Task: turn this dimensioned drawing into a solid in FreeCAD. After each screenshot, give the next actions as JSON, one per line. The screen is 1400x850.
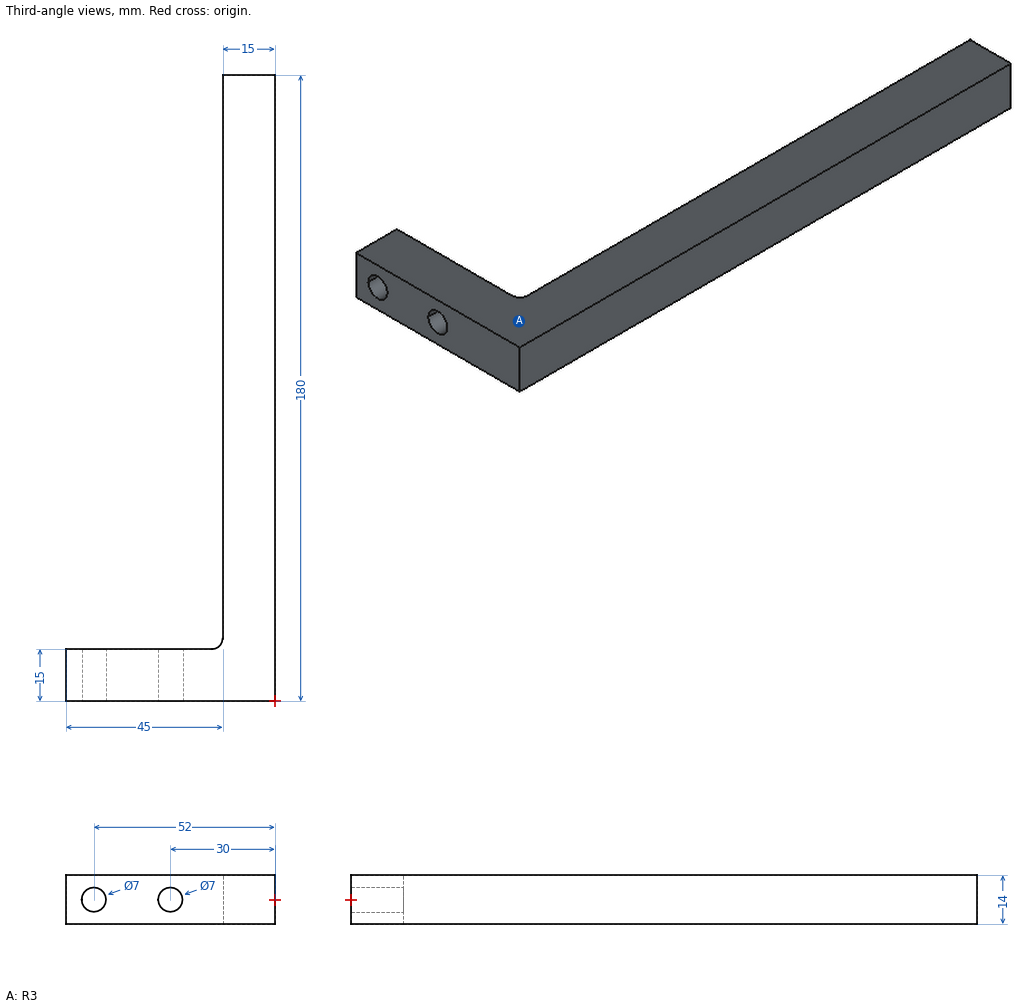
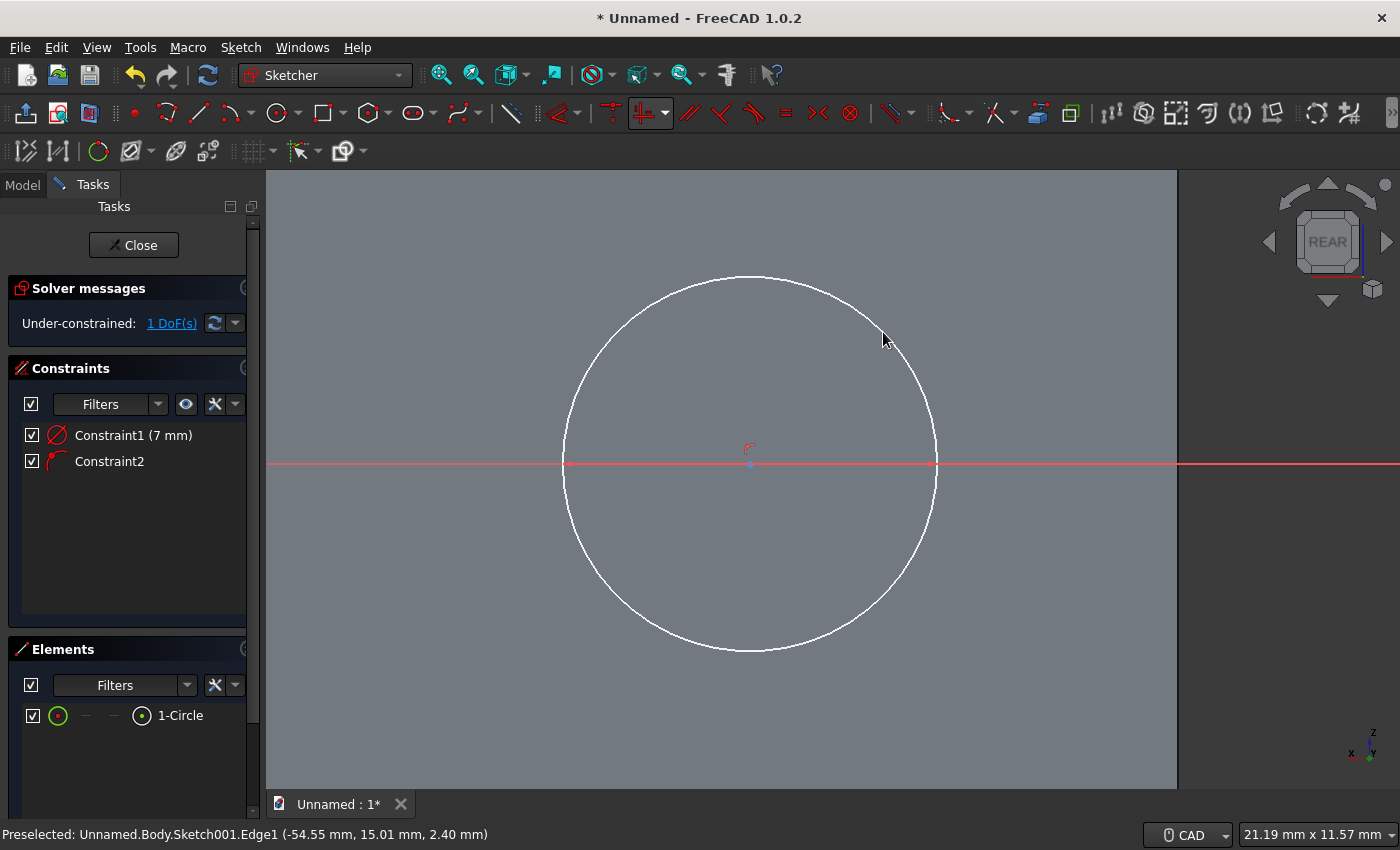
{"action": "left_click", "coordinate": [750, 464]}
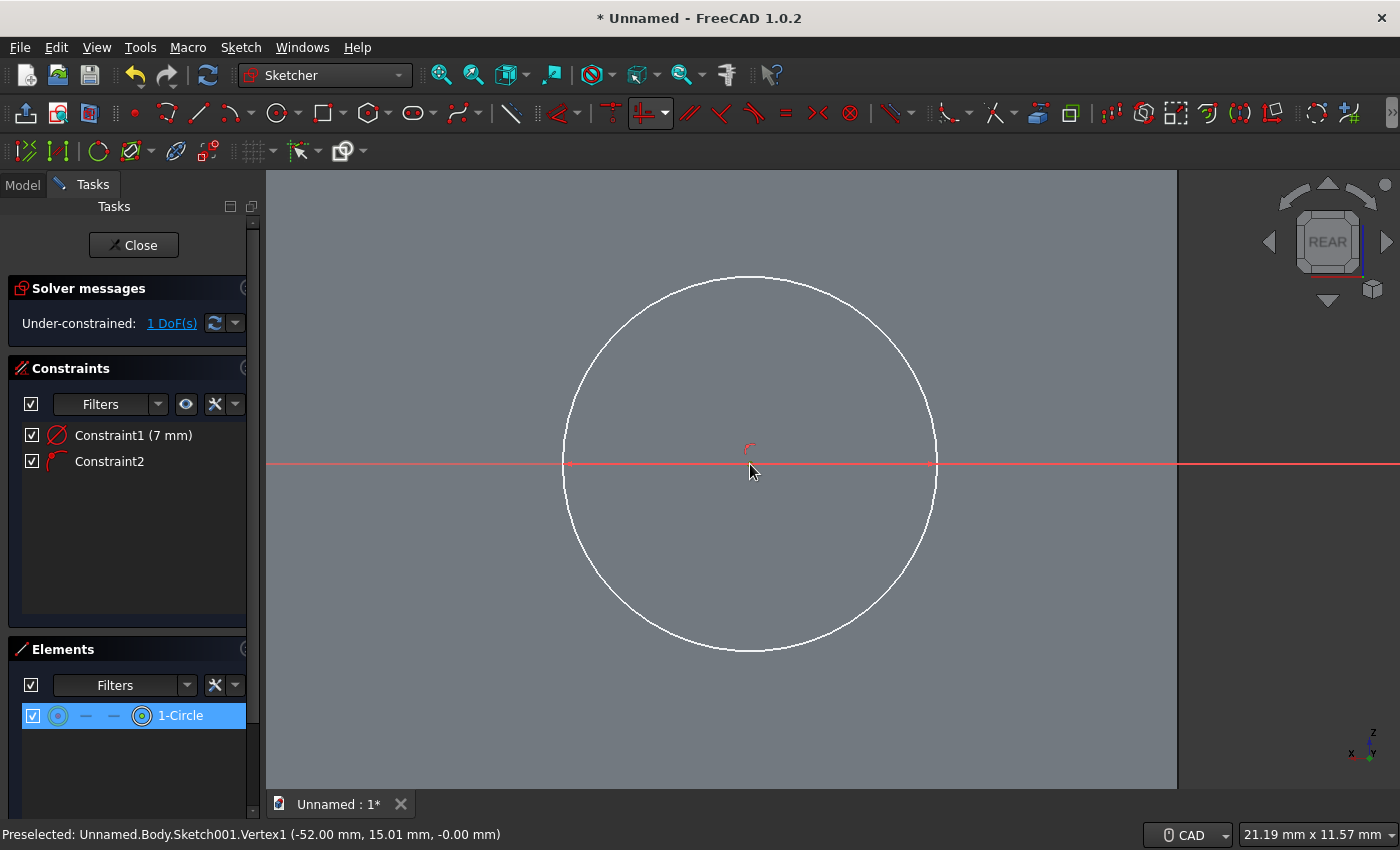
{"action": "left_click", "coordinate": [580, 114]}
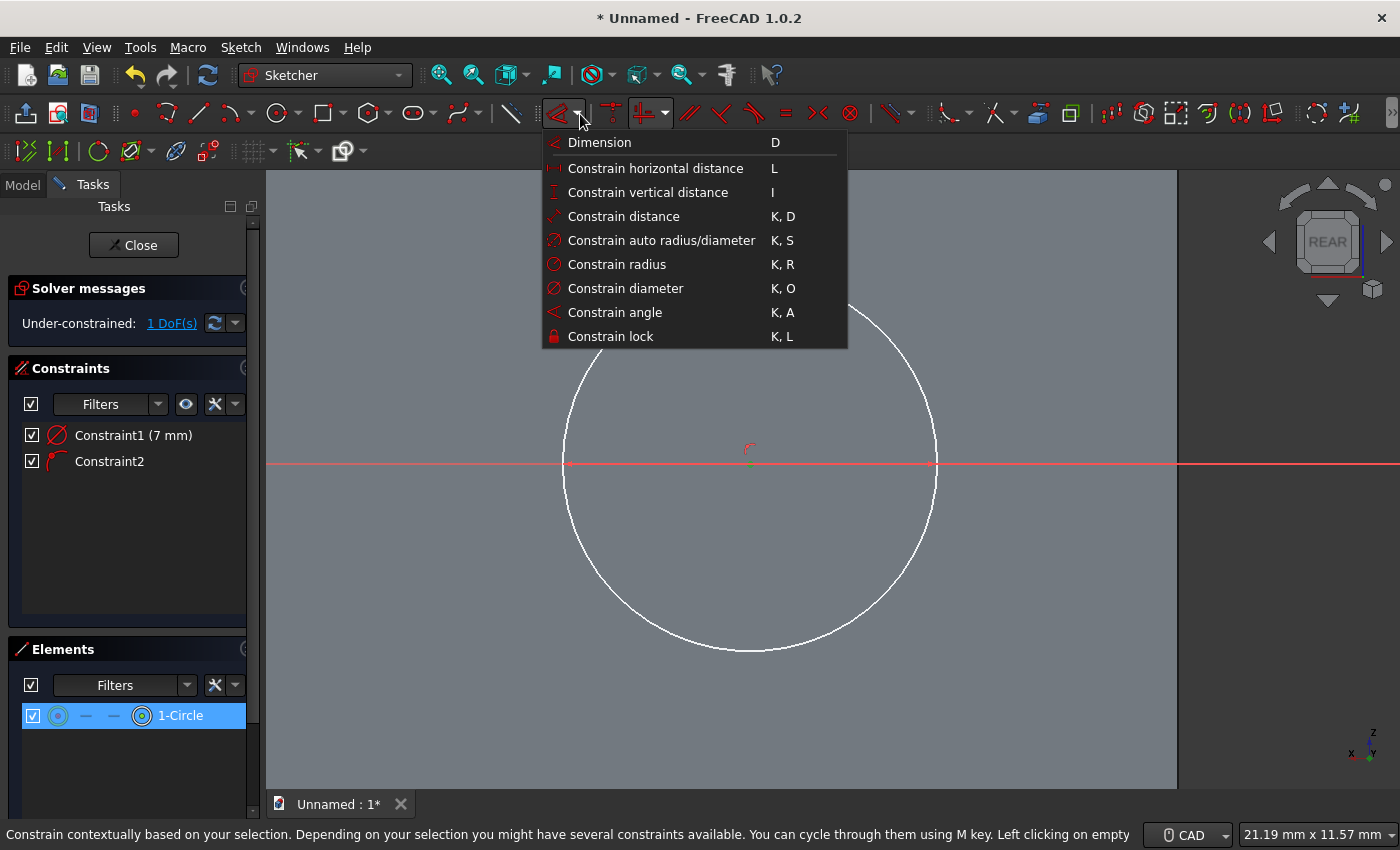
{"action": "left_click", "coordinate": [695, 168]}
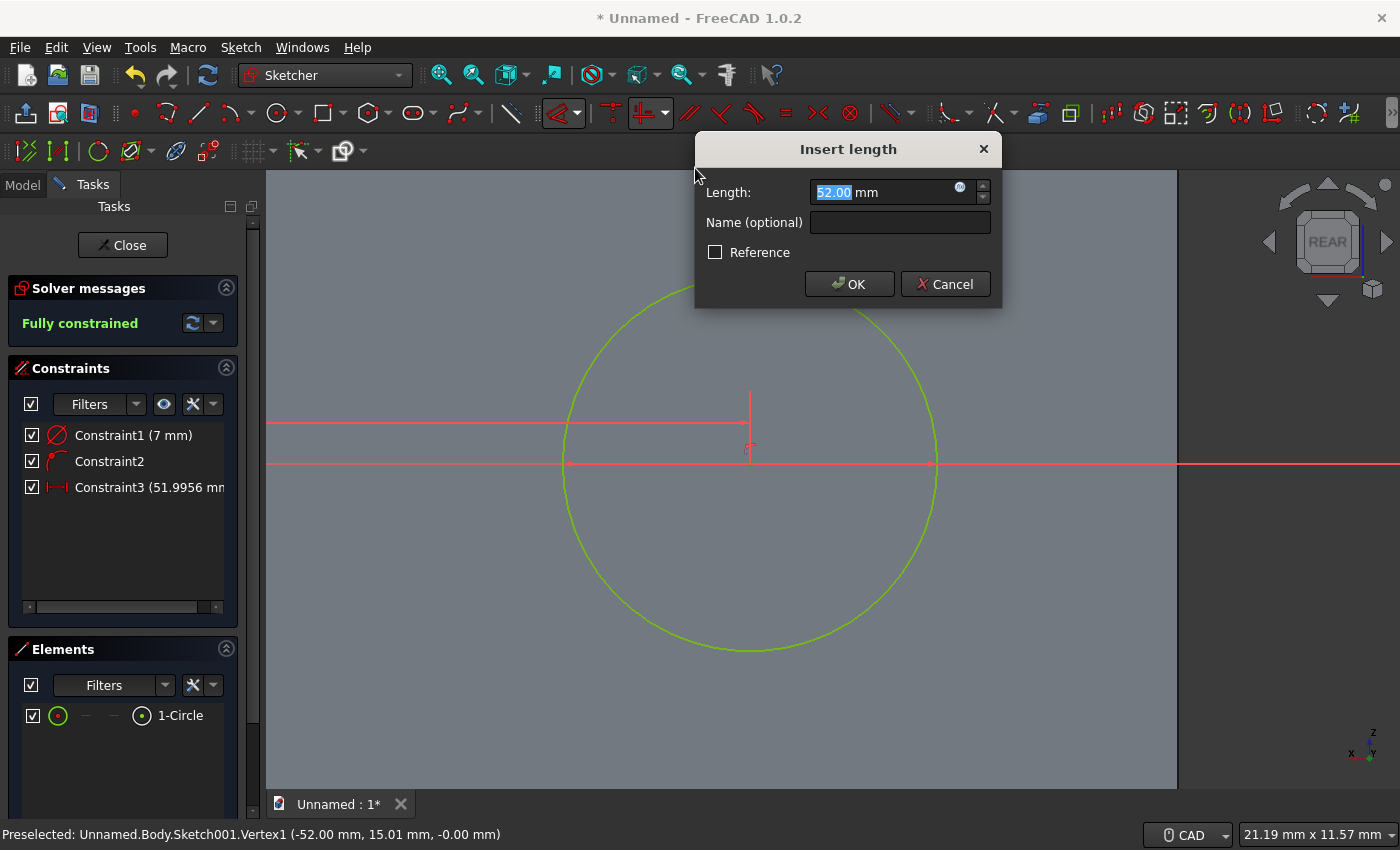
{"action": "type", "text": "52"}
{"action": "key", "text": "Return"}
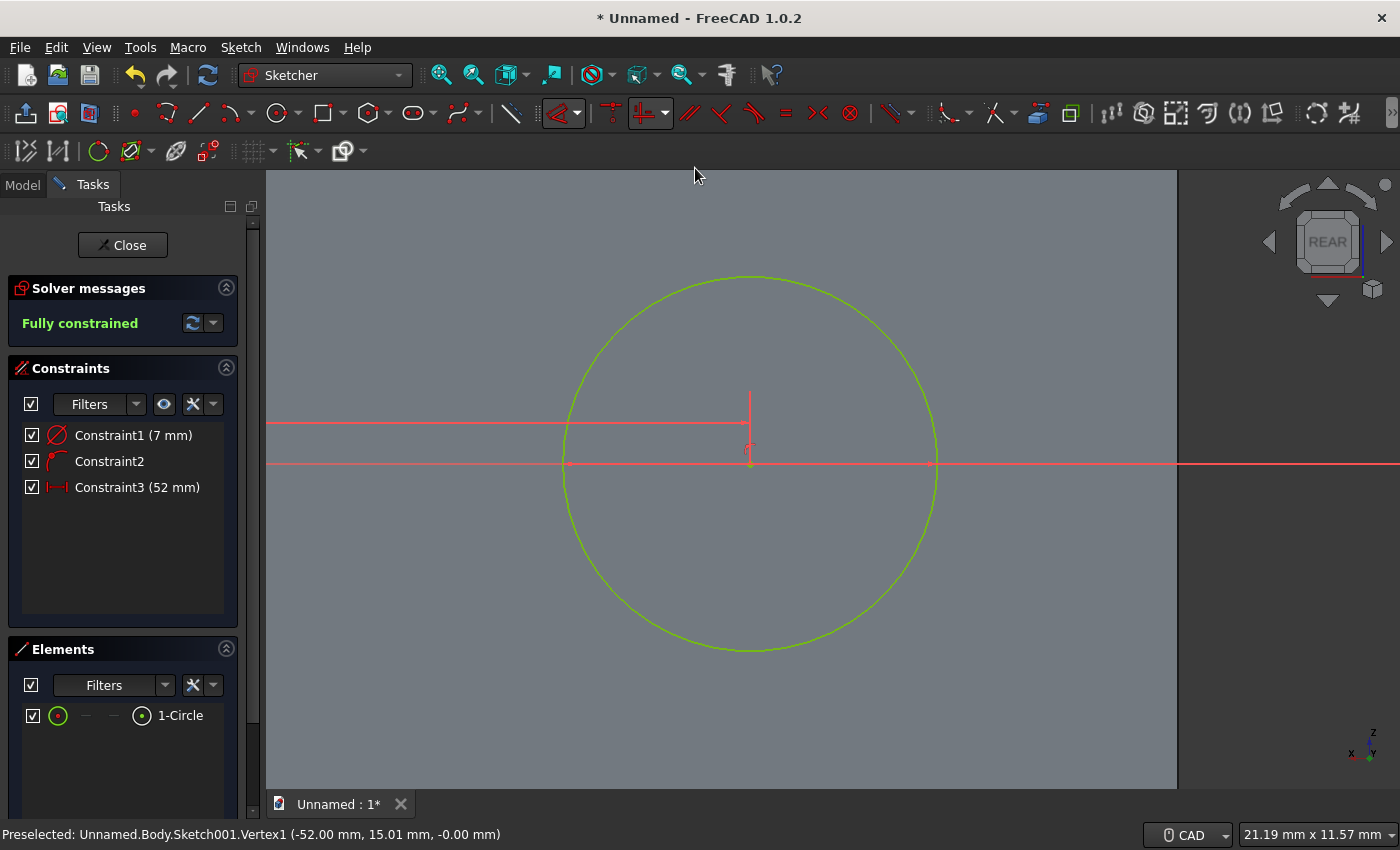
{"action": "left_click", "coordinate": [123, 245]}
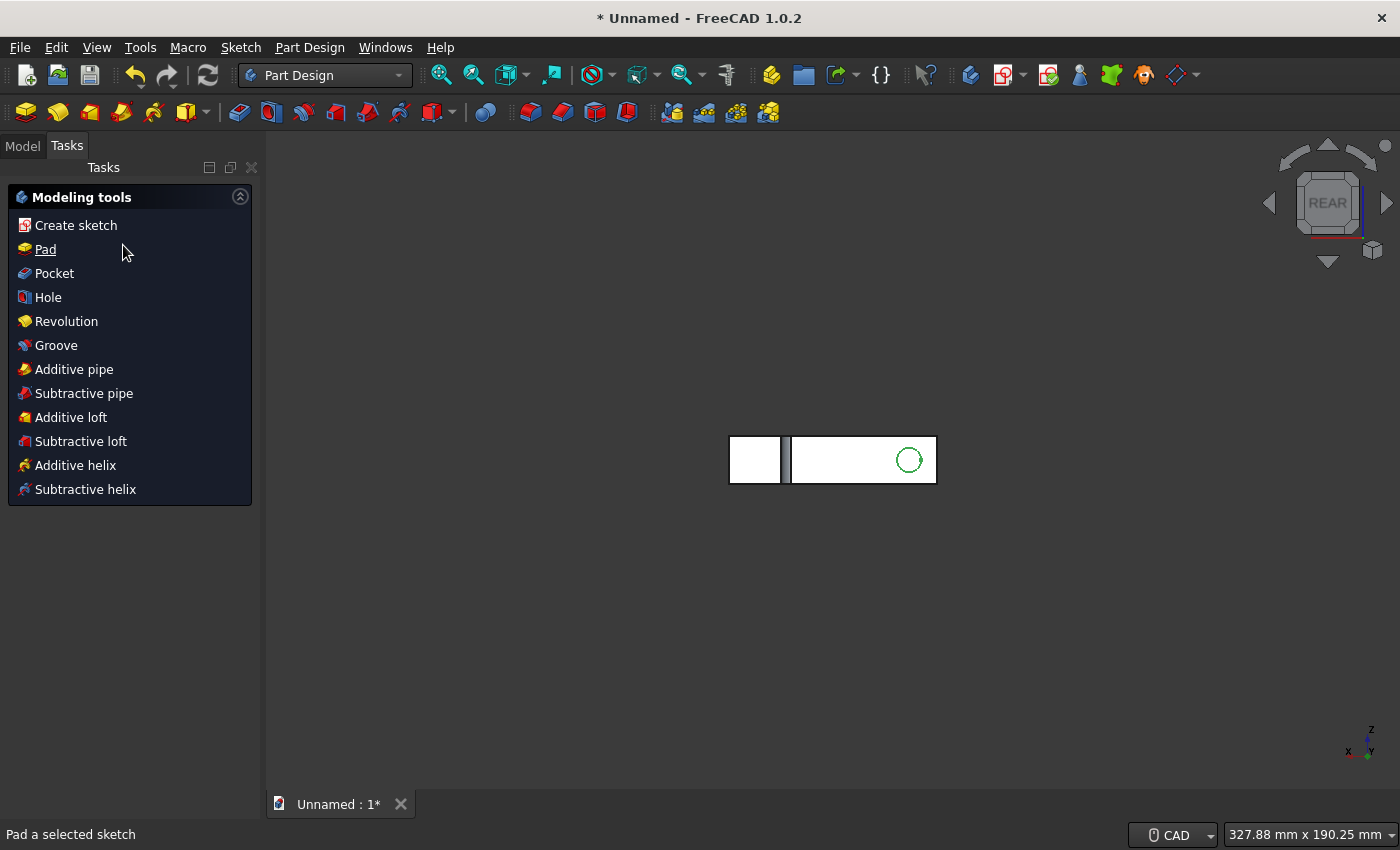
{"action": "left_click", "coordinate": [240, 112]}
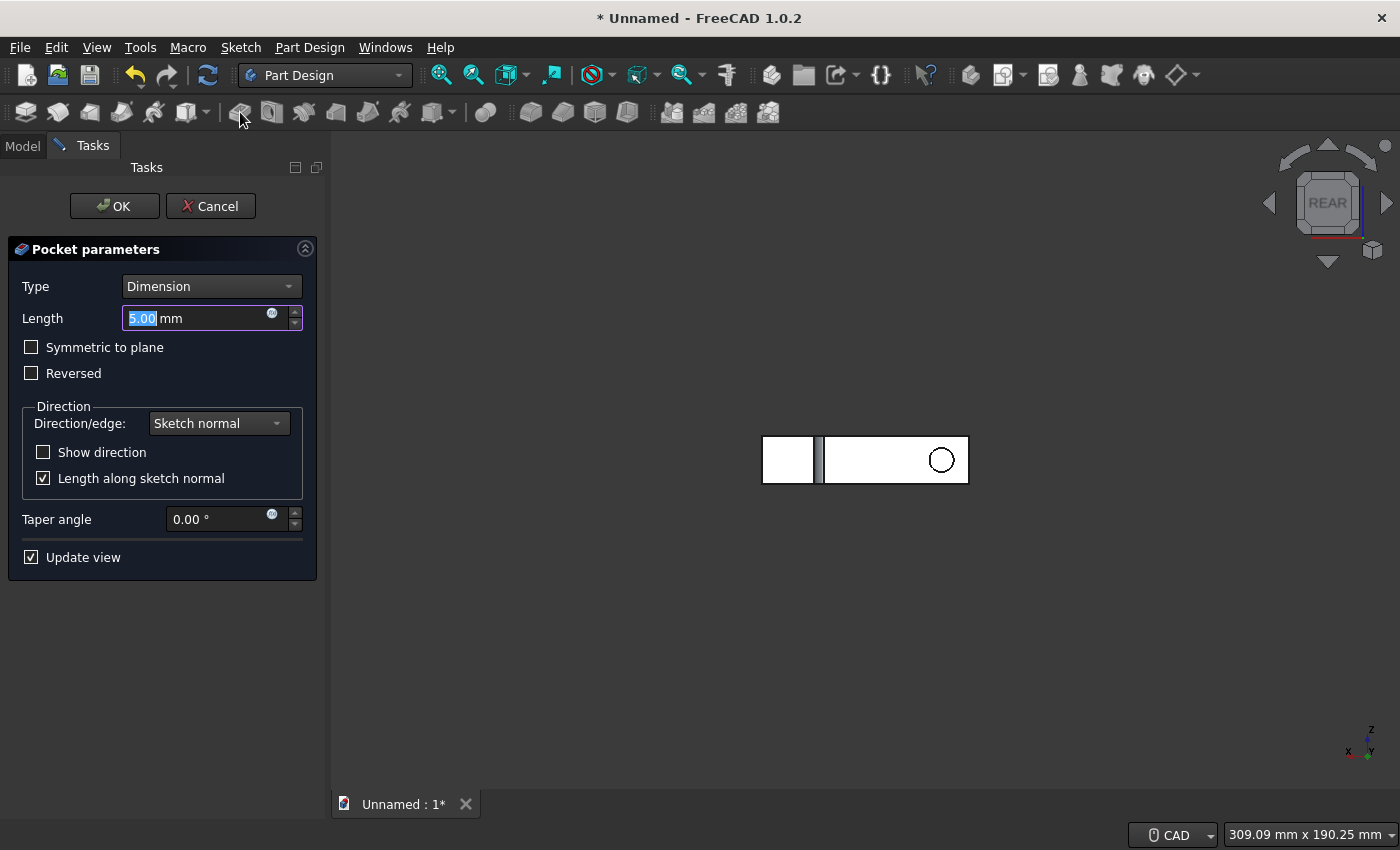
{"action": "left_click", "coordinate": [212, 286]}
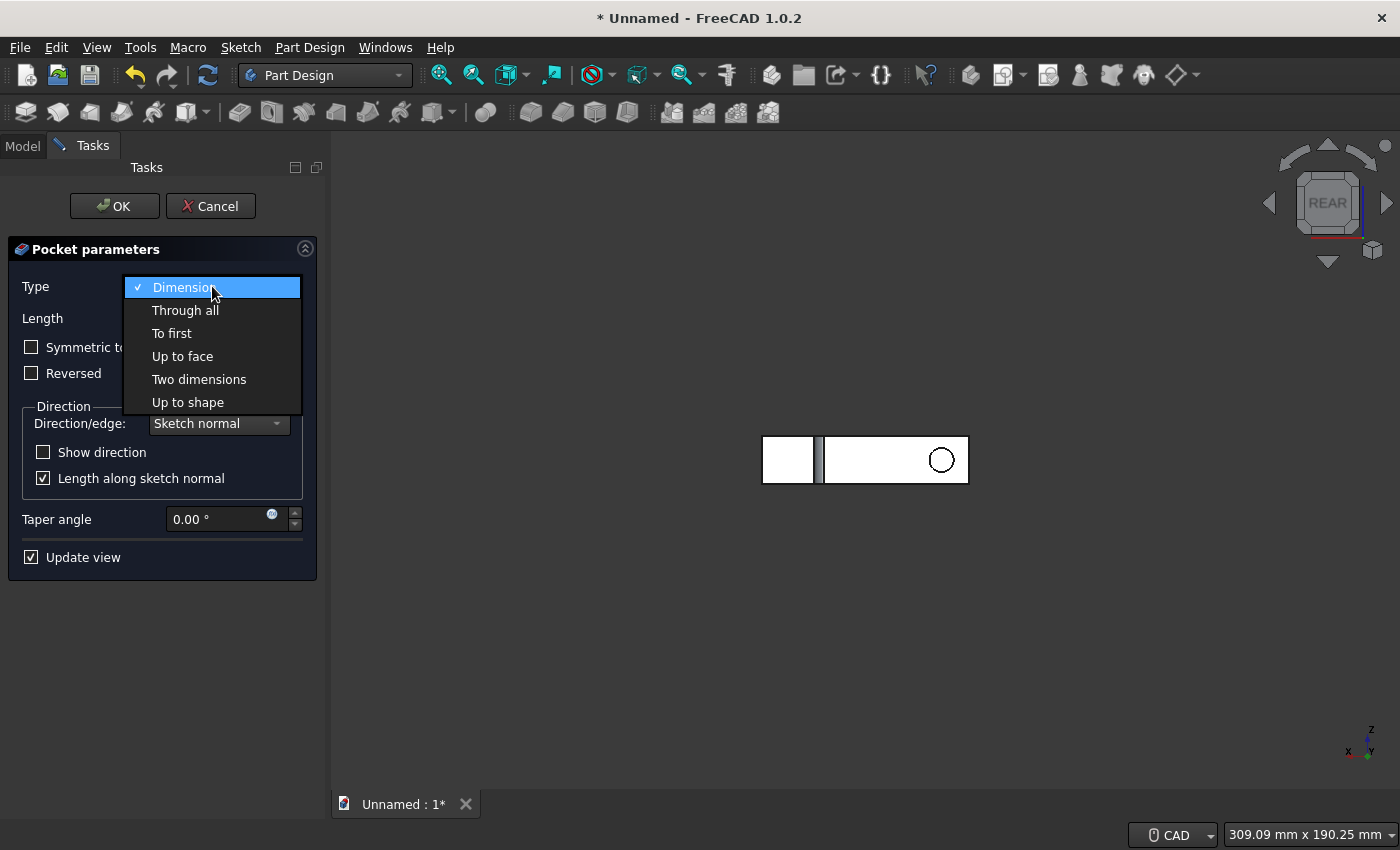
{"action": "left_click", "coordinate": [212, 334]}